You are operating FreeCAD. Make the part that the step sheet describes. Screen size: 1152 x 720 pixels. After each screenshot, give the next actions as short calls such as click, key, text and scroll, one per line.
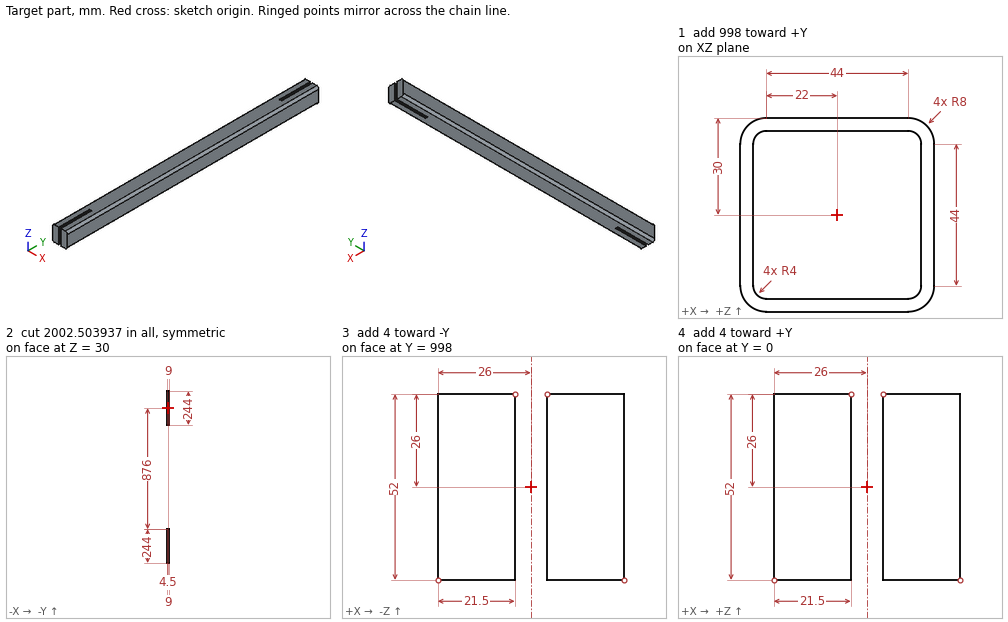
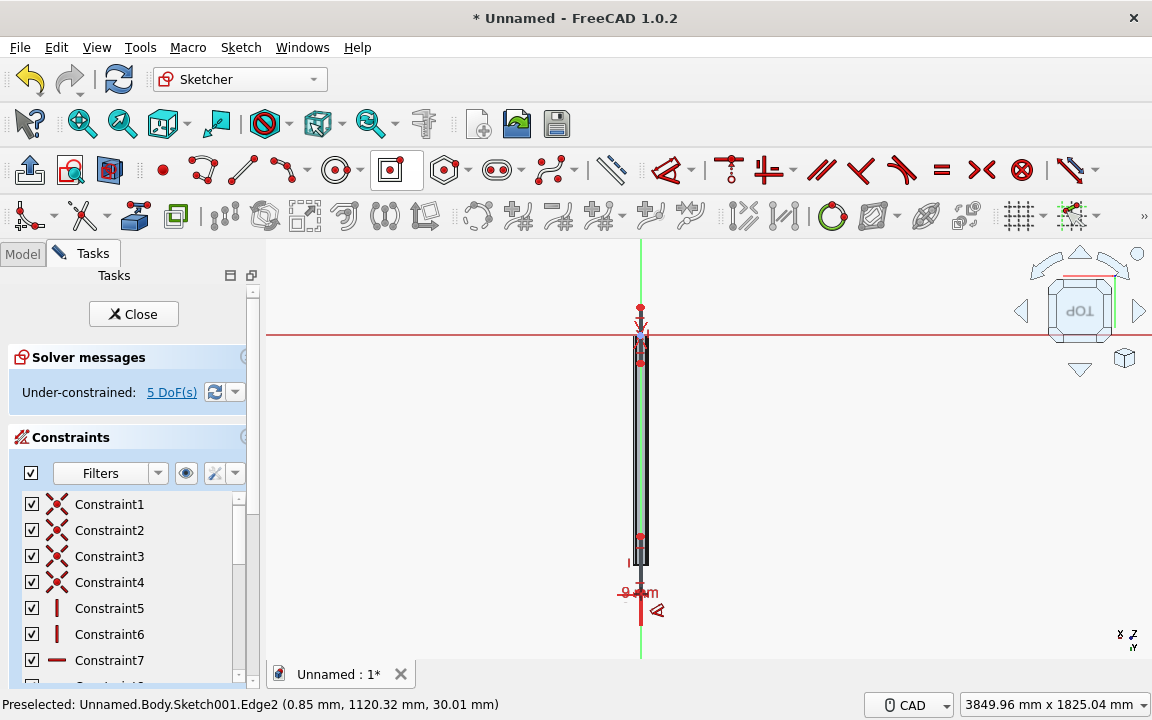
scroll(641, 363, up, 15)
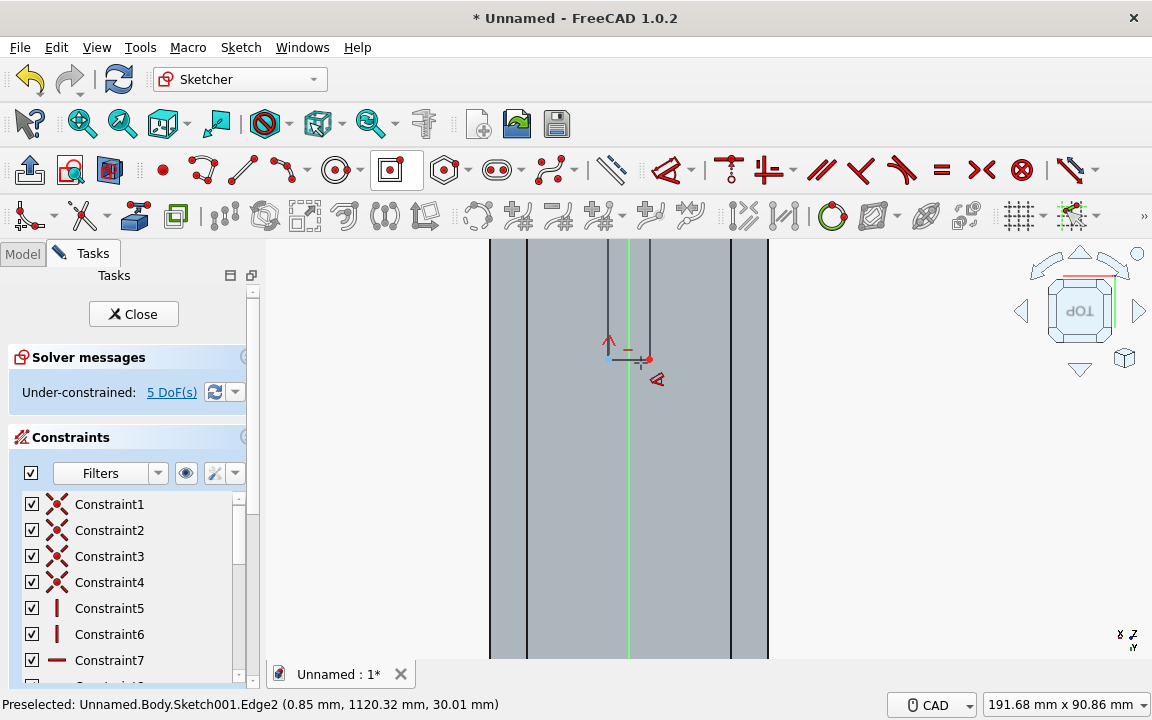
click(629, 360)
click(615, 394)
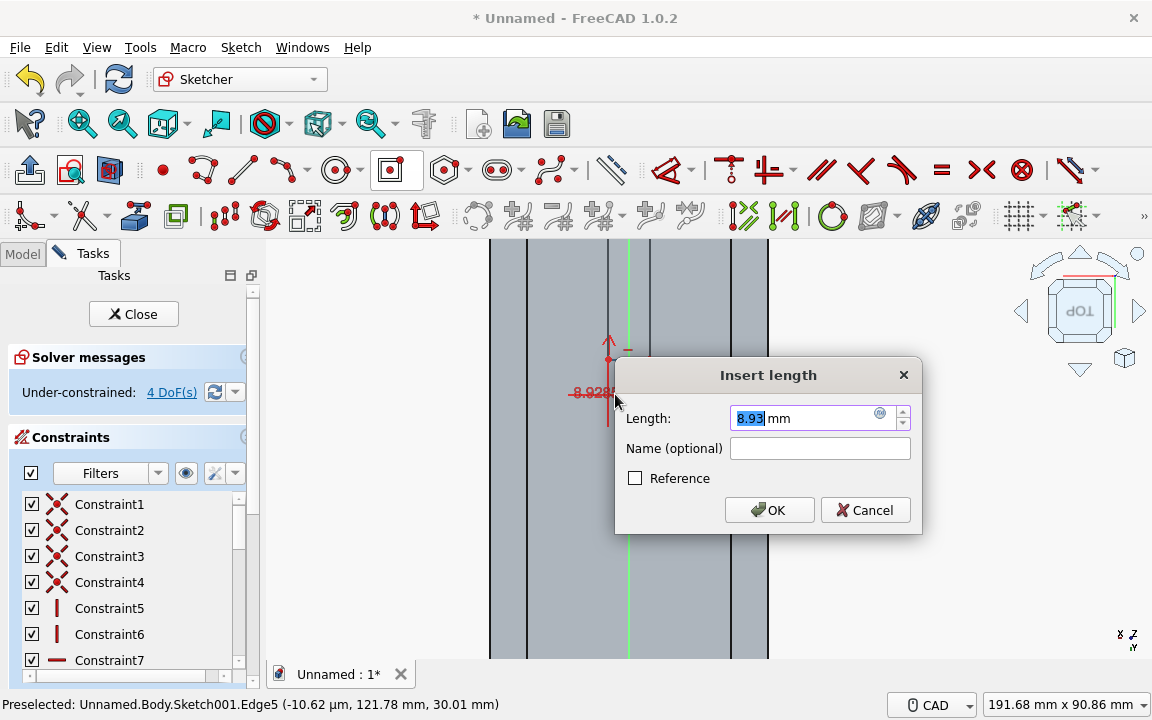
text(9)
key(Return)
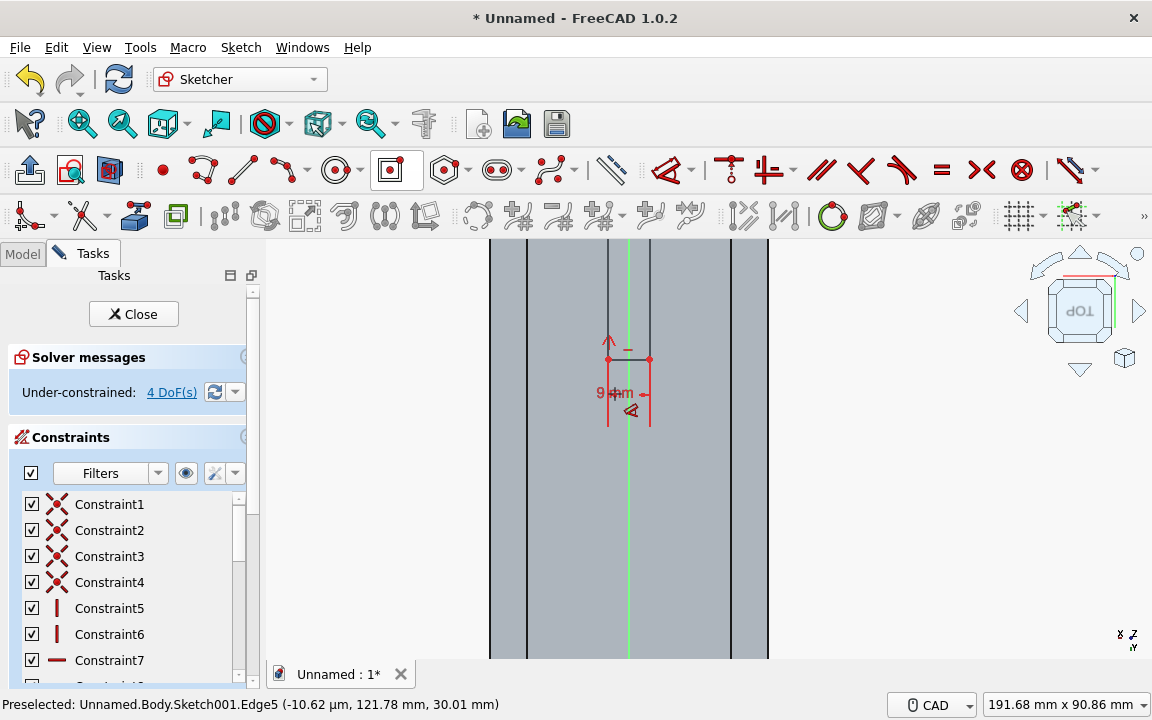
scroll(641, 362, down, 15)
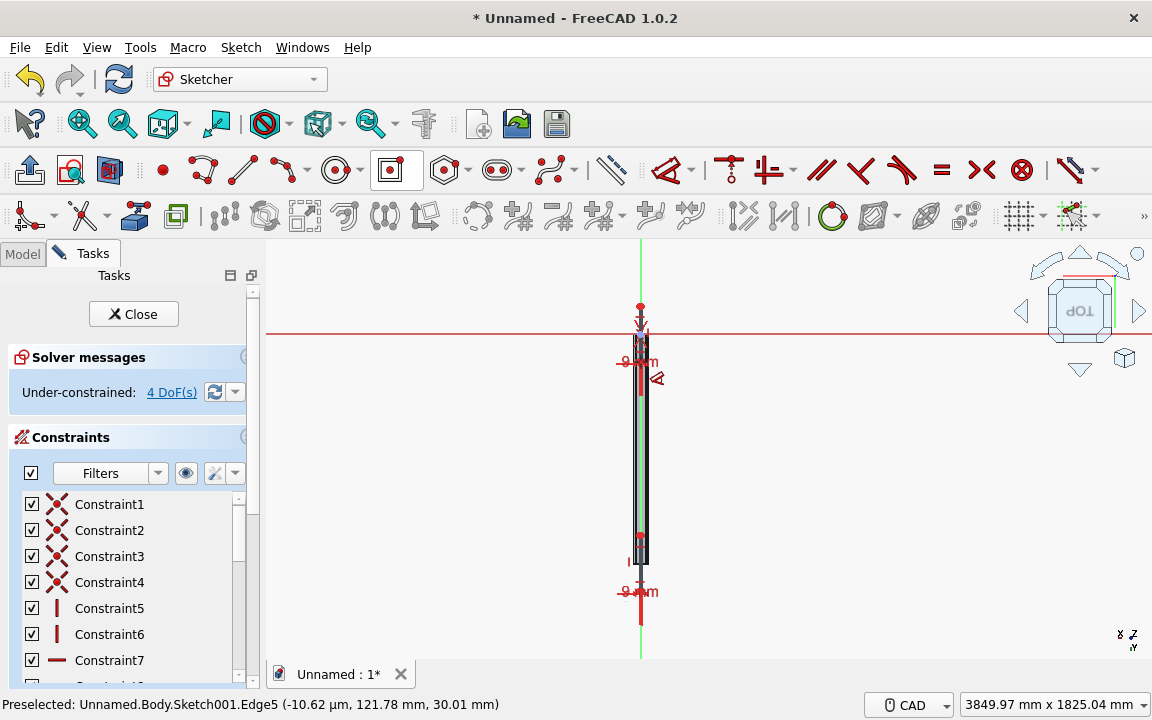
scroll(640, 553, up, 13)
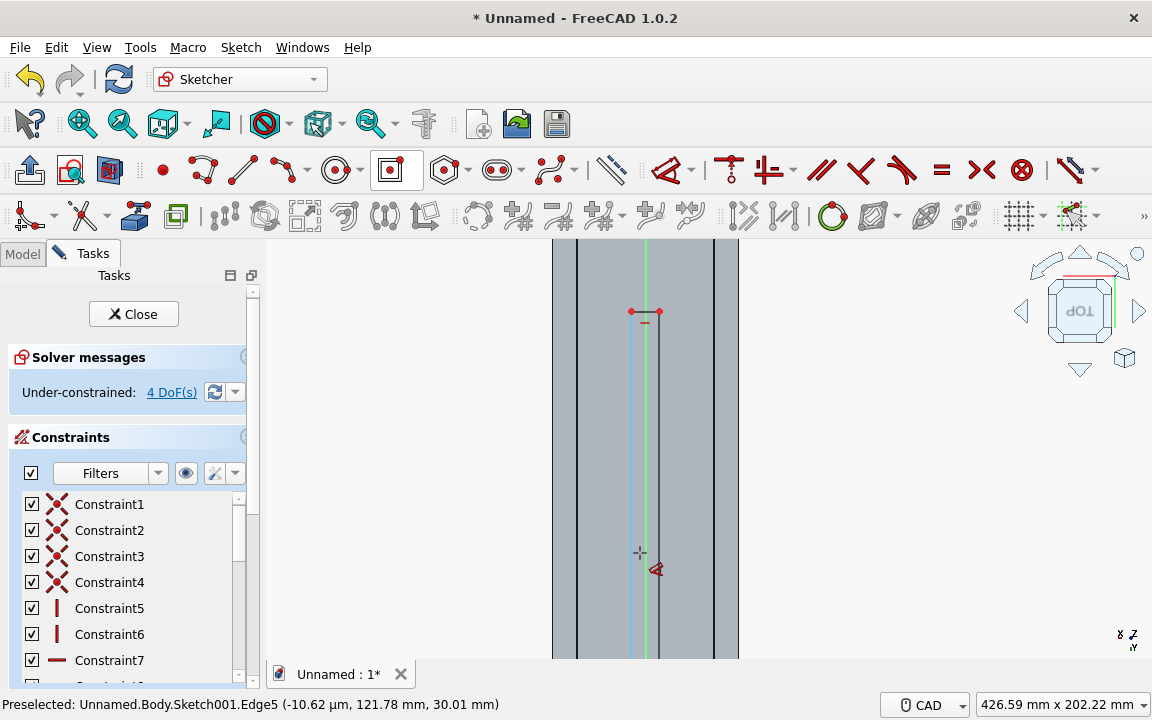
click(631, 539)
click(597, 471)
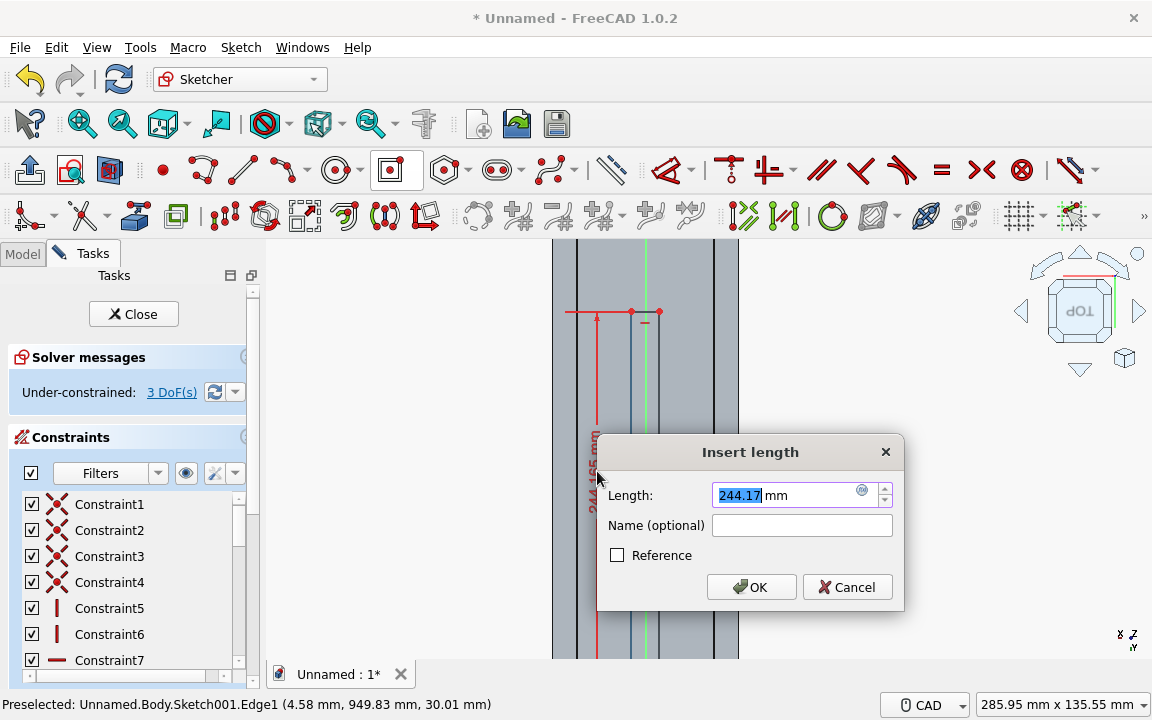
text(244)
key(Return)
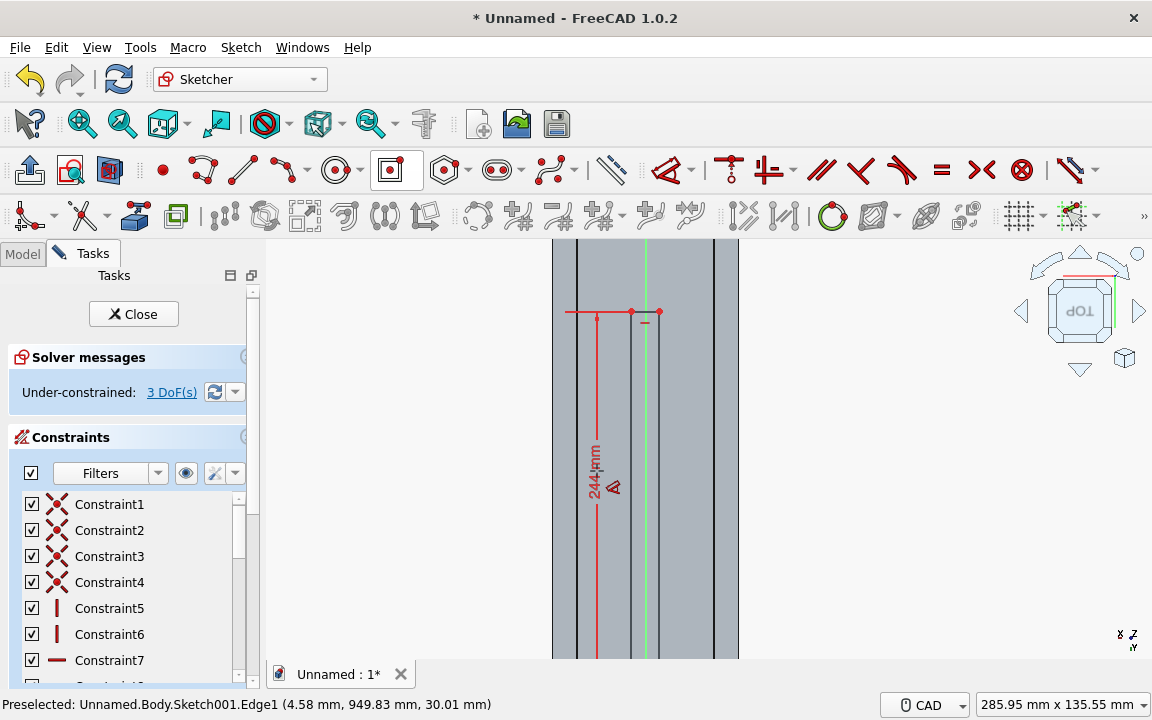
scroll(640, 534, down, 14)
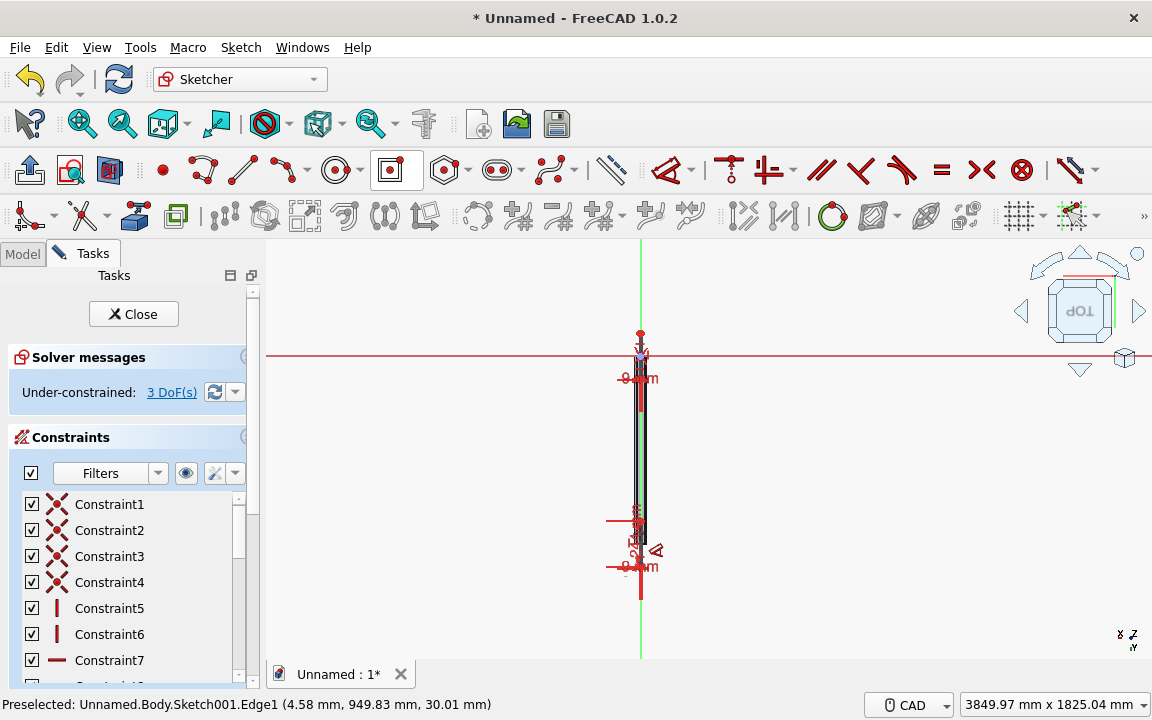
scroll(642, 365, up, 14)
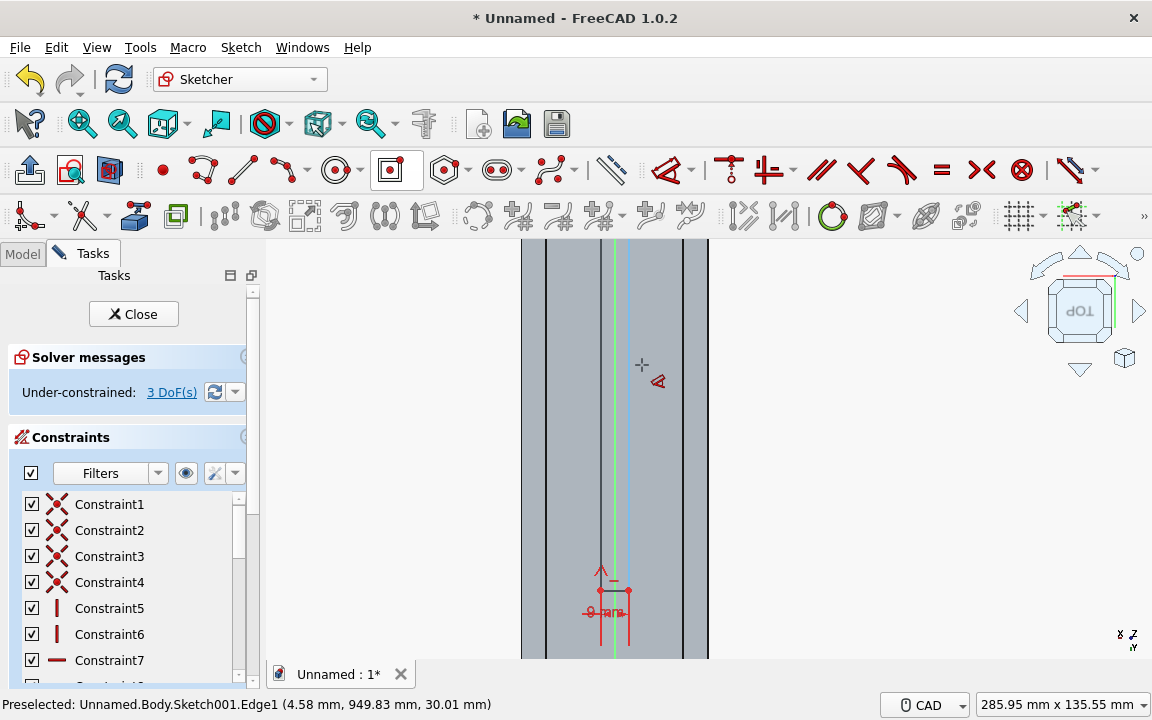
click(629, 364)
click(663, 429)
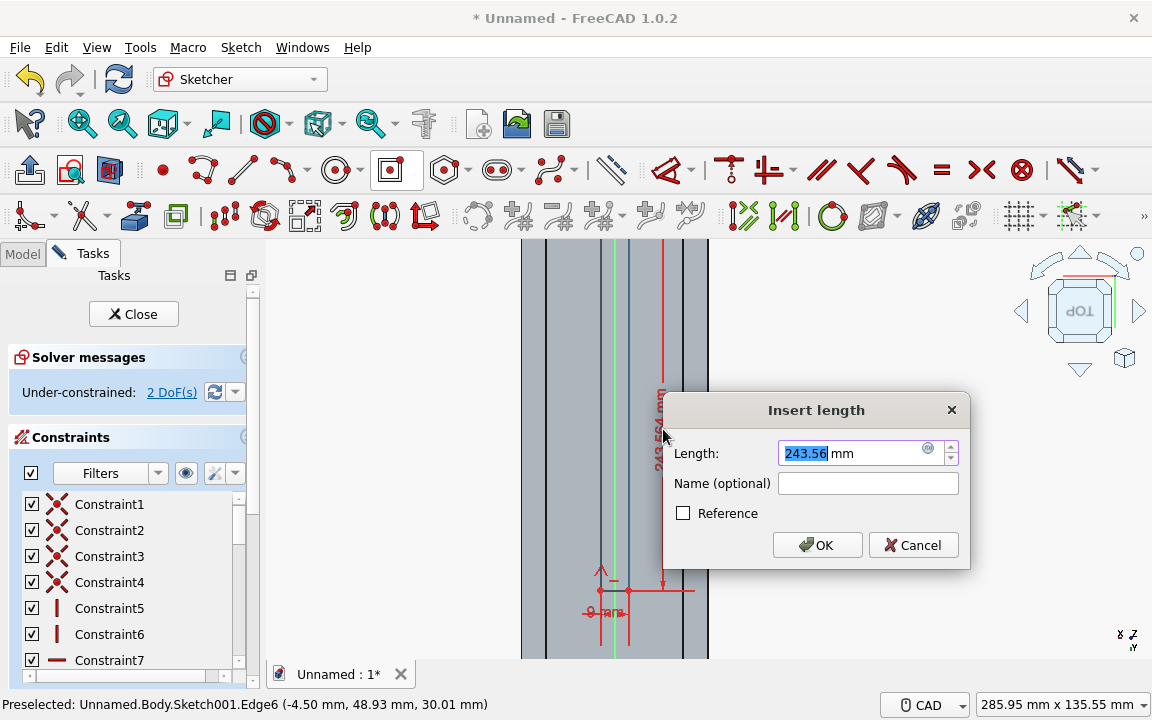
text(244)
key(Return)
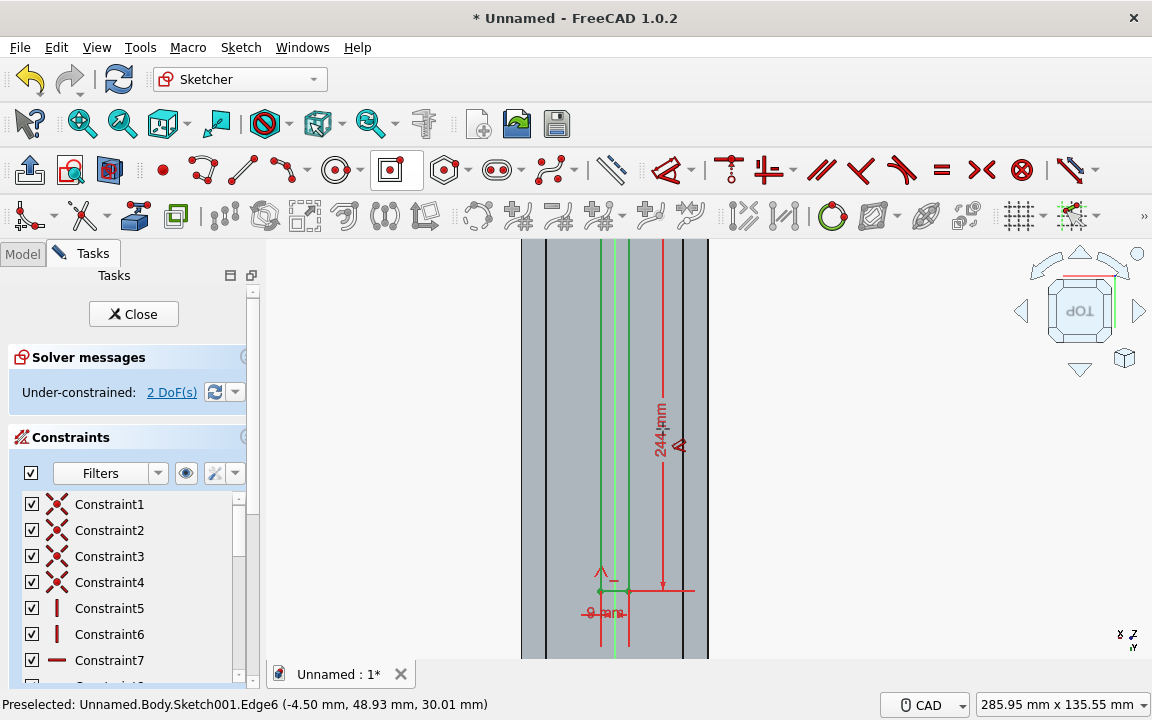
scroll(642, 364, down, 14)